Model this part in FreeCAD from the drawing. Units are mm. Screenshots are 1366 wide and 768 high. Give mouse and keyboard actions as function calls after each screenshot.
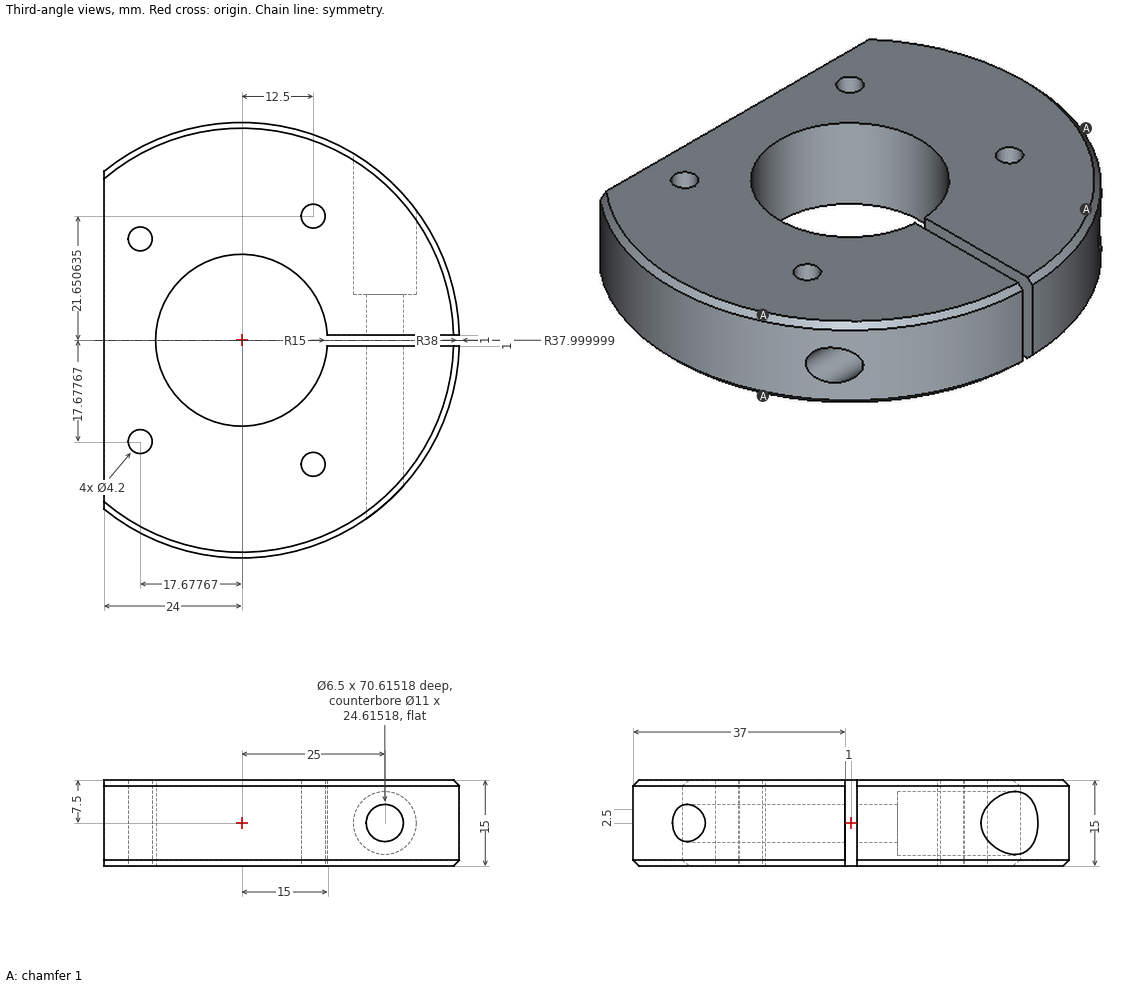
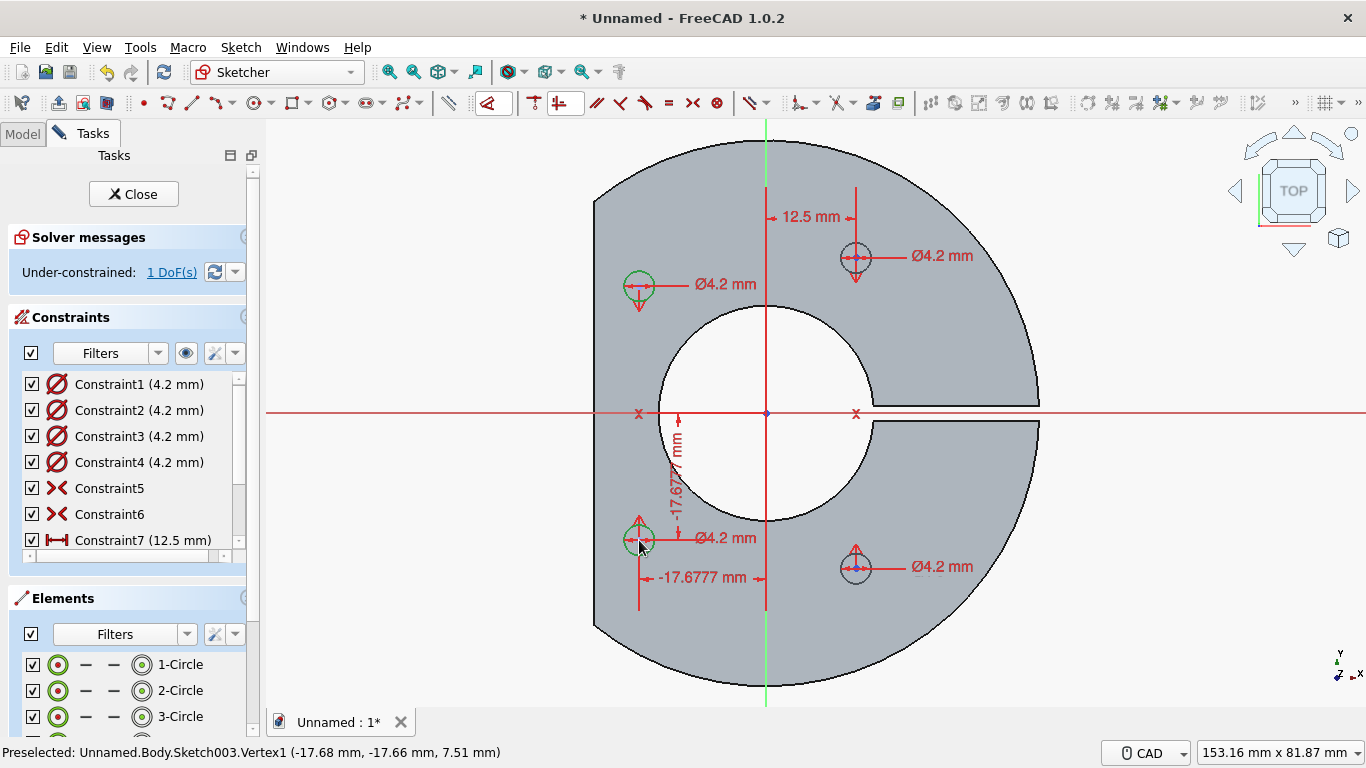
click(856, 258)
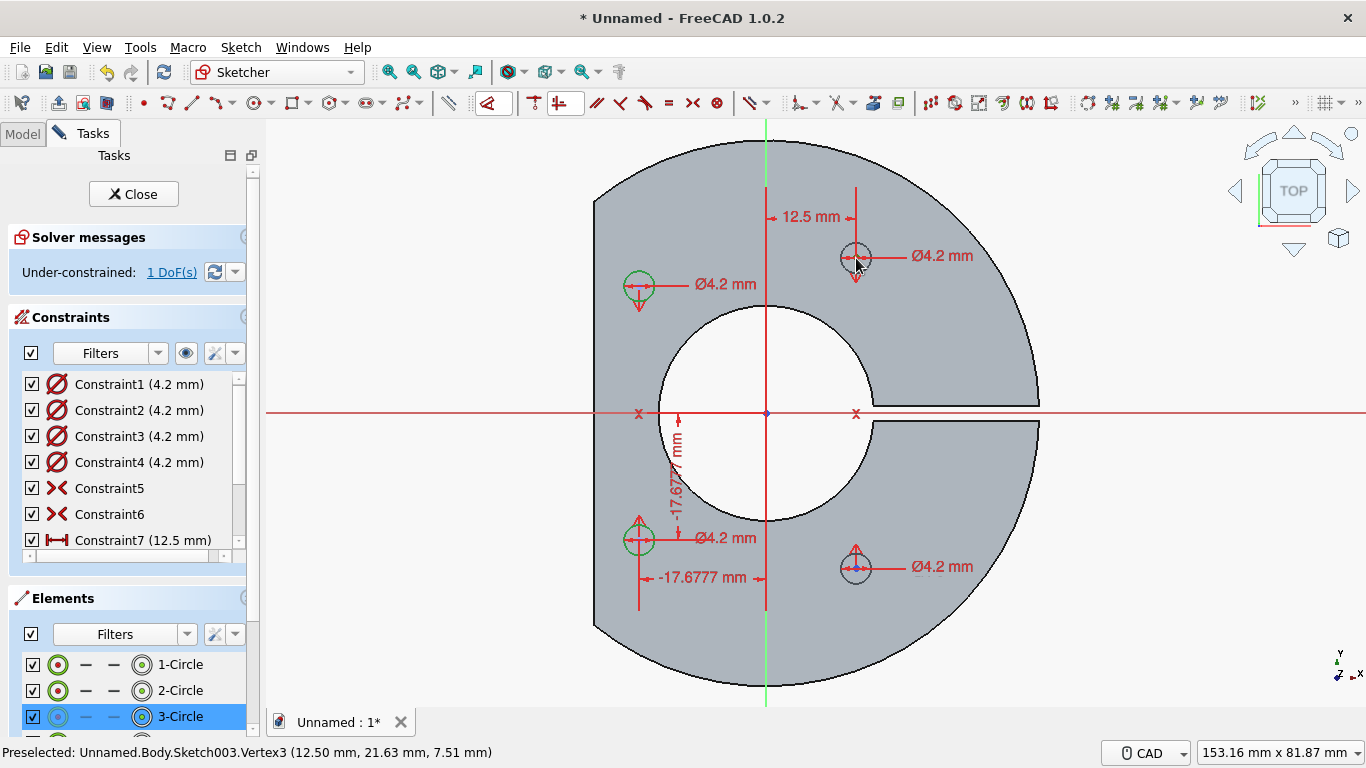
click(506, 104)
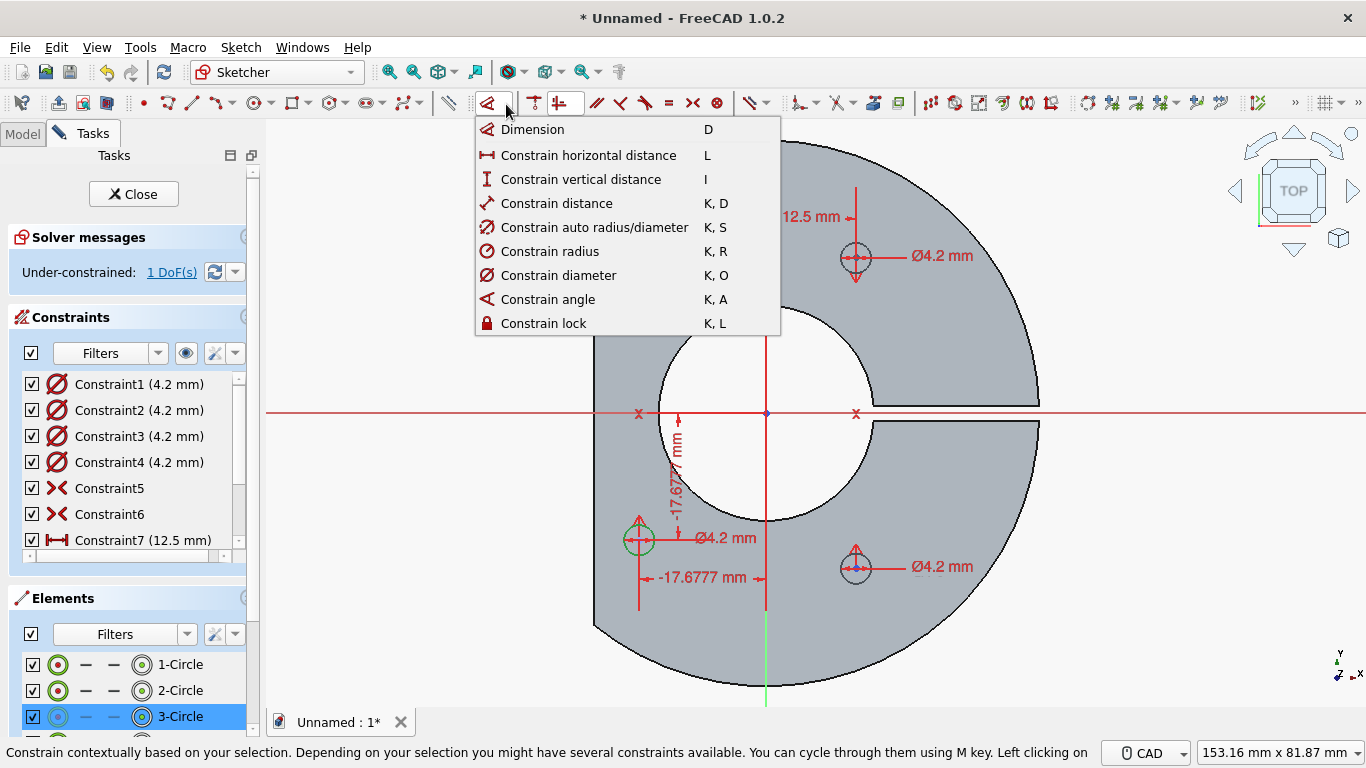
click(628, 179)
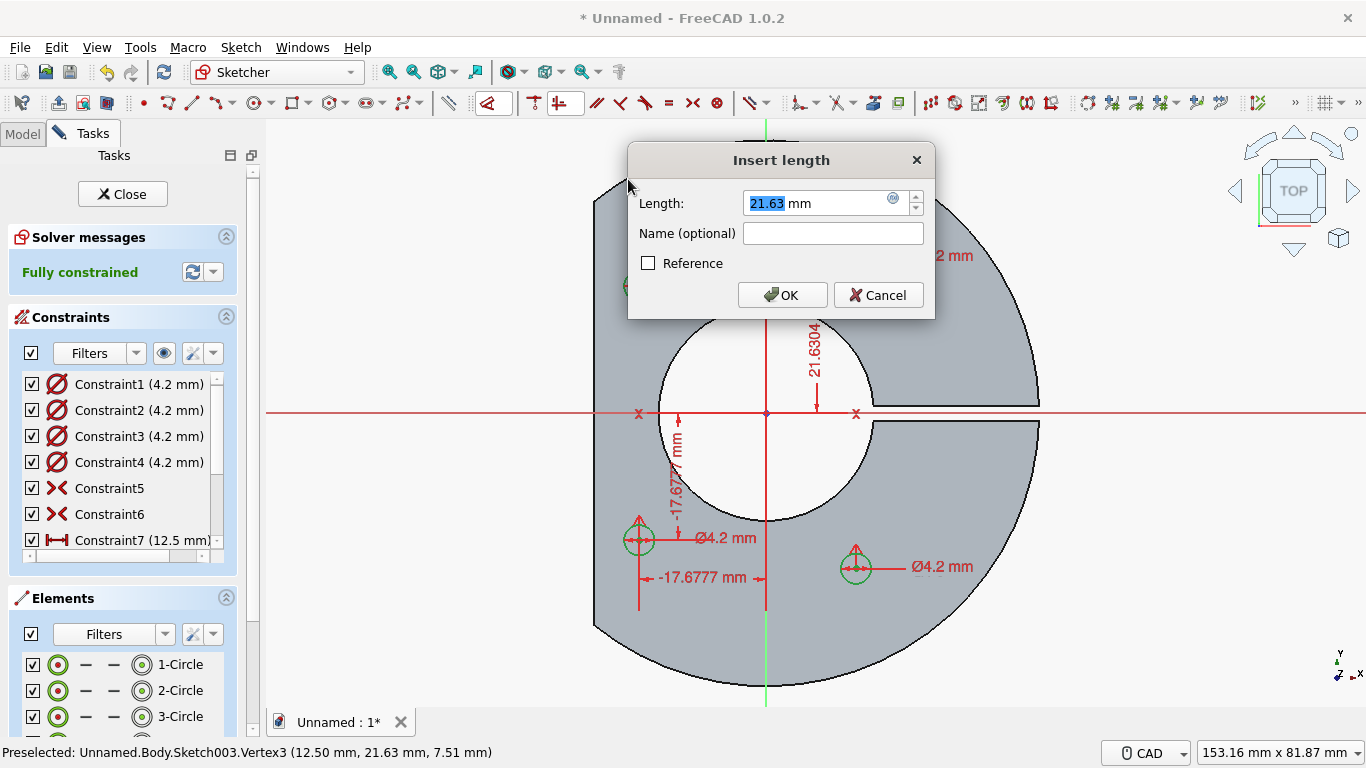
text(21.650635)
key(Return)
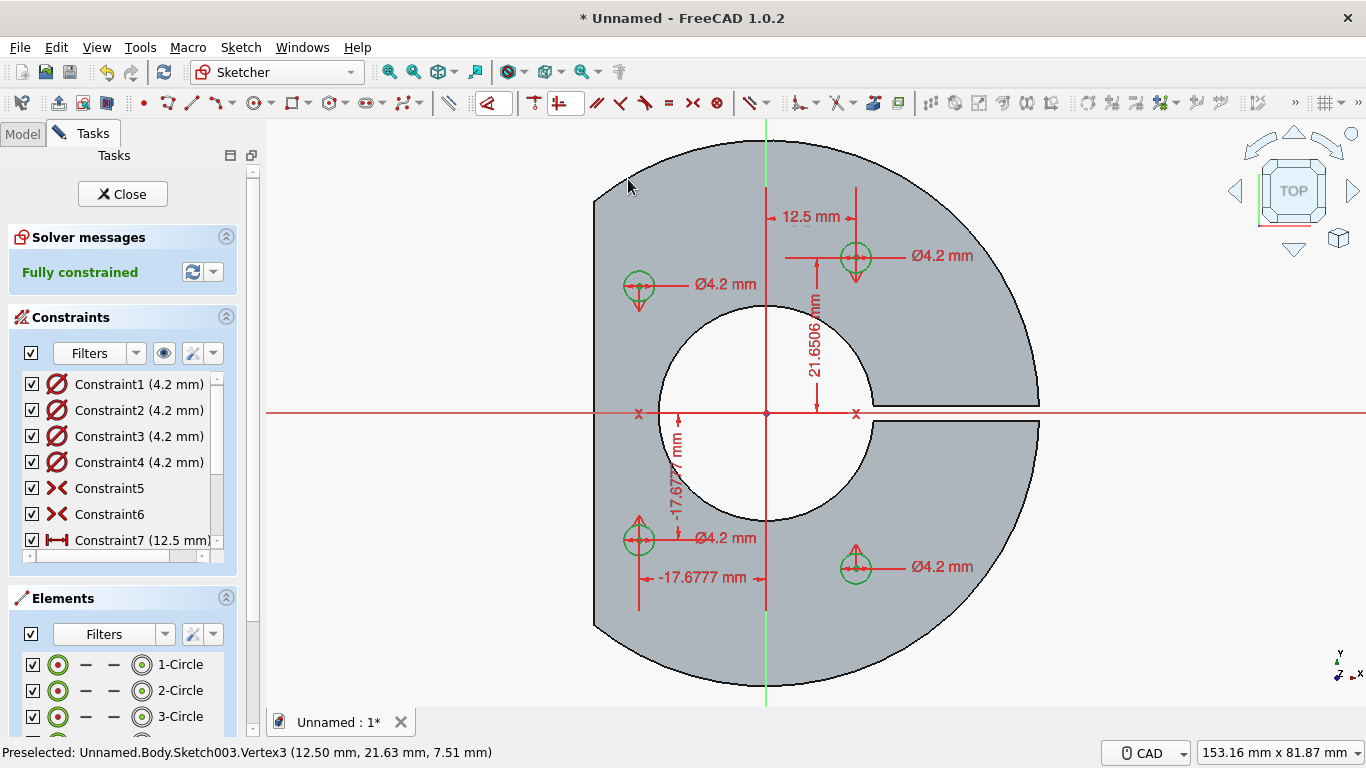
click(123, 194)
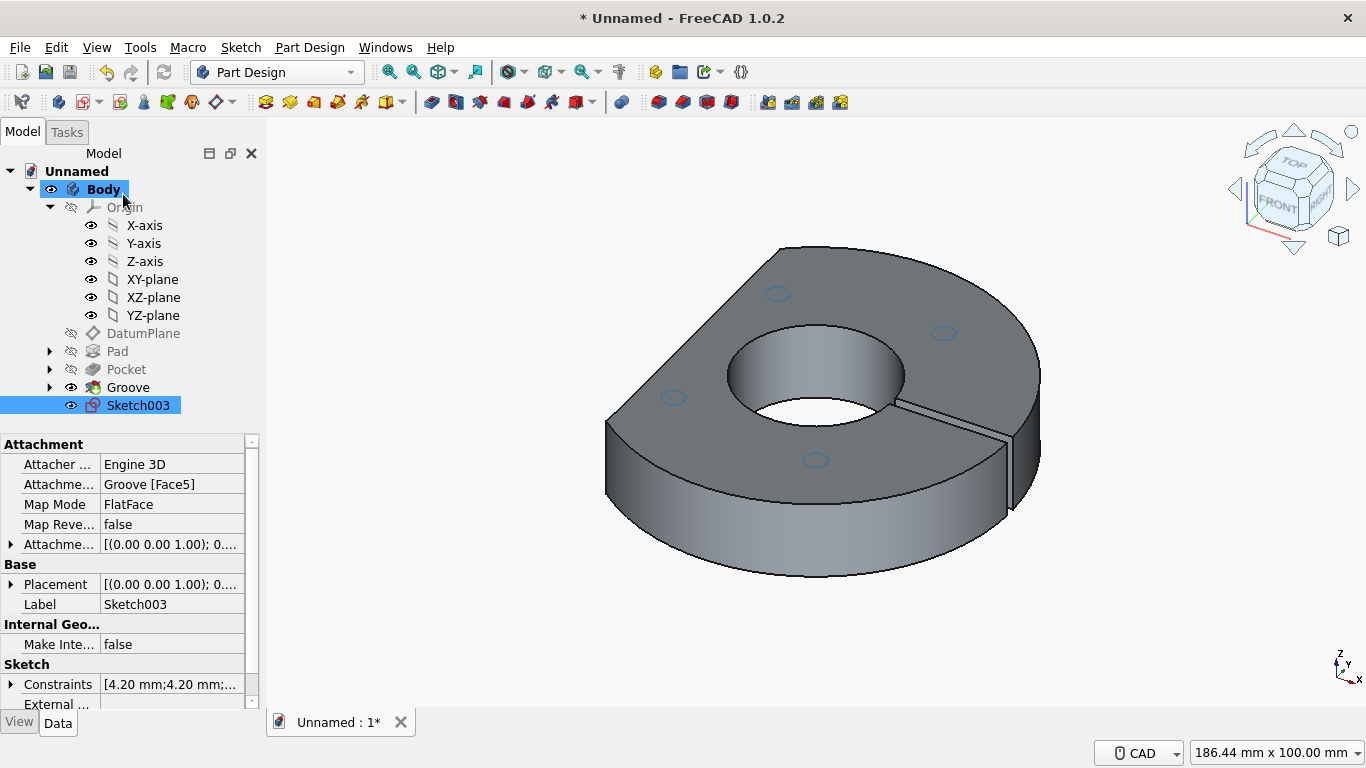
click(432, 102)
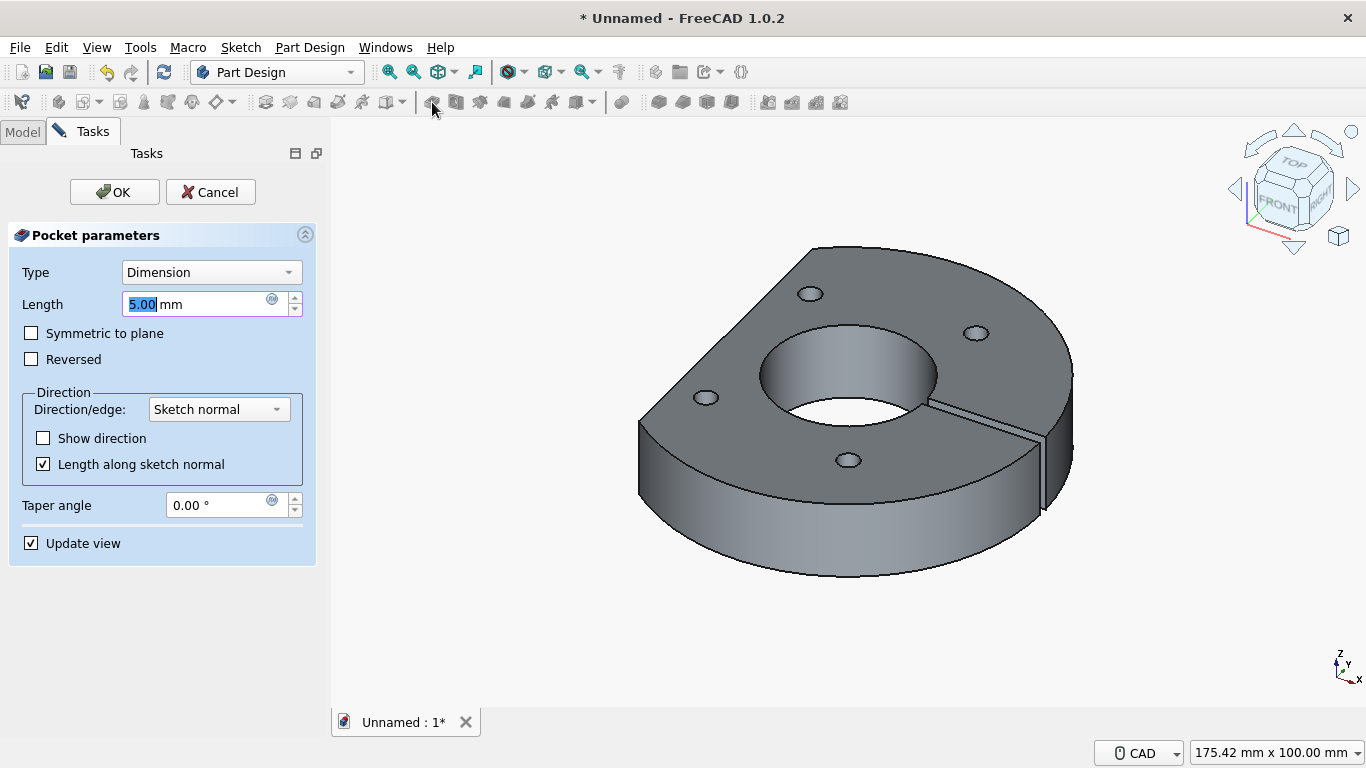
click(212, 272)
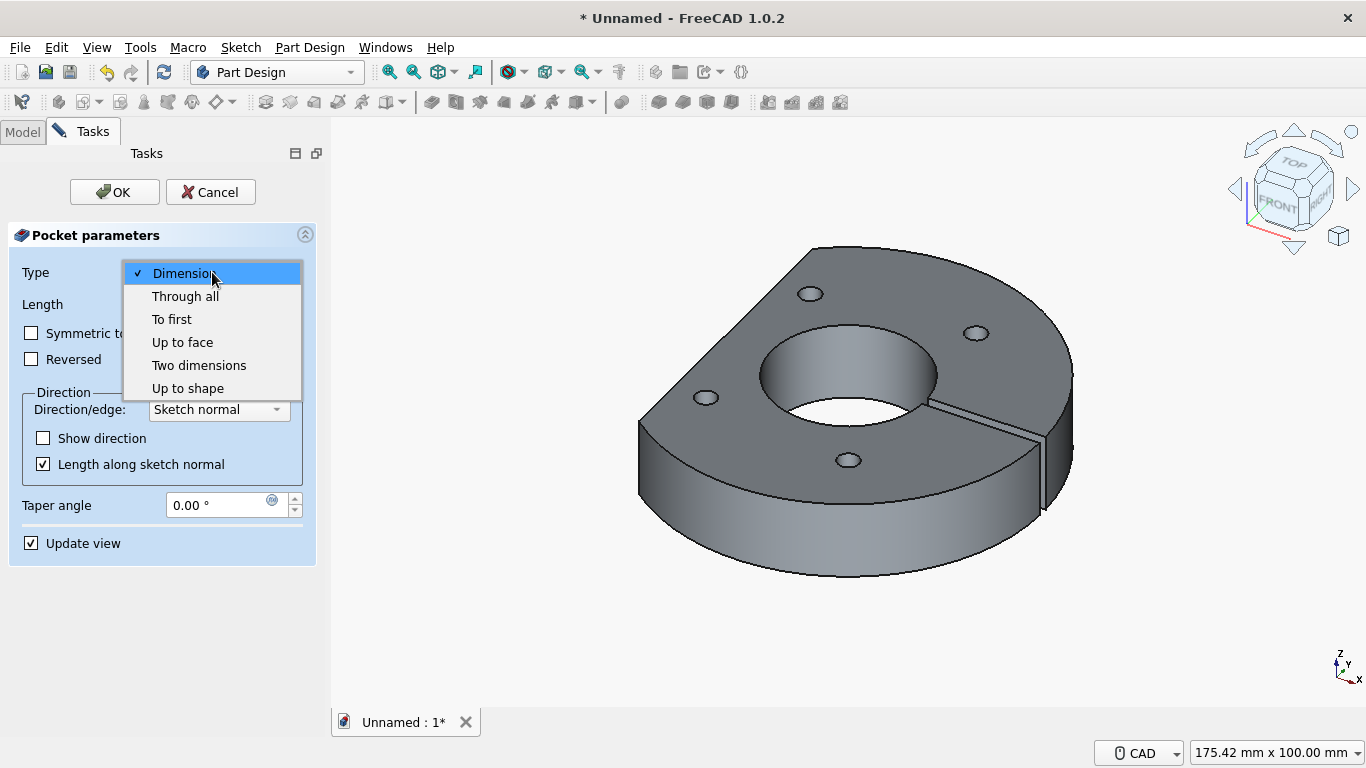
click(212, 296)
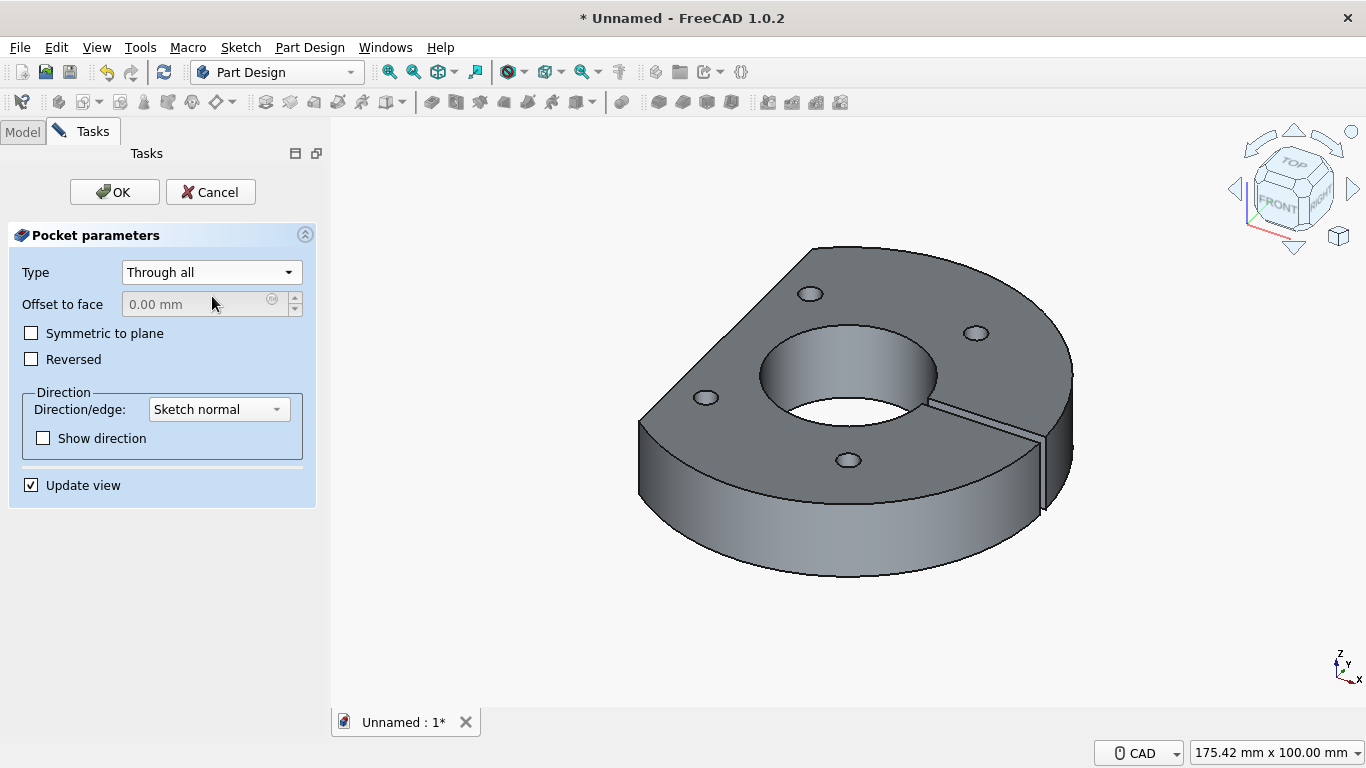
click(115, 192)